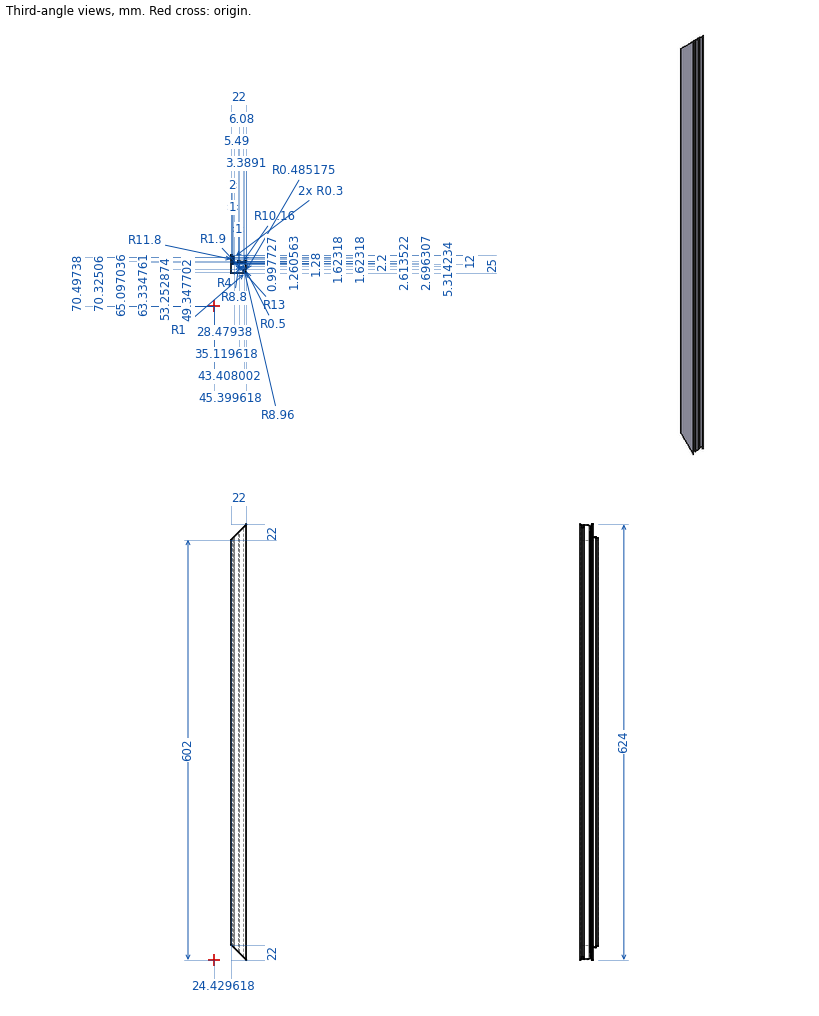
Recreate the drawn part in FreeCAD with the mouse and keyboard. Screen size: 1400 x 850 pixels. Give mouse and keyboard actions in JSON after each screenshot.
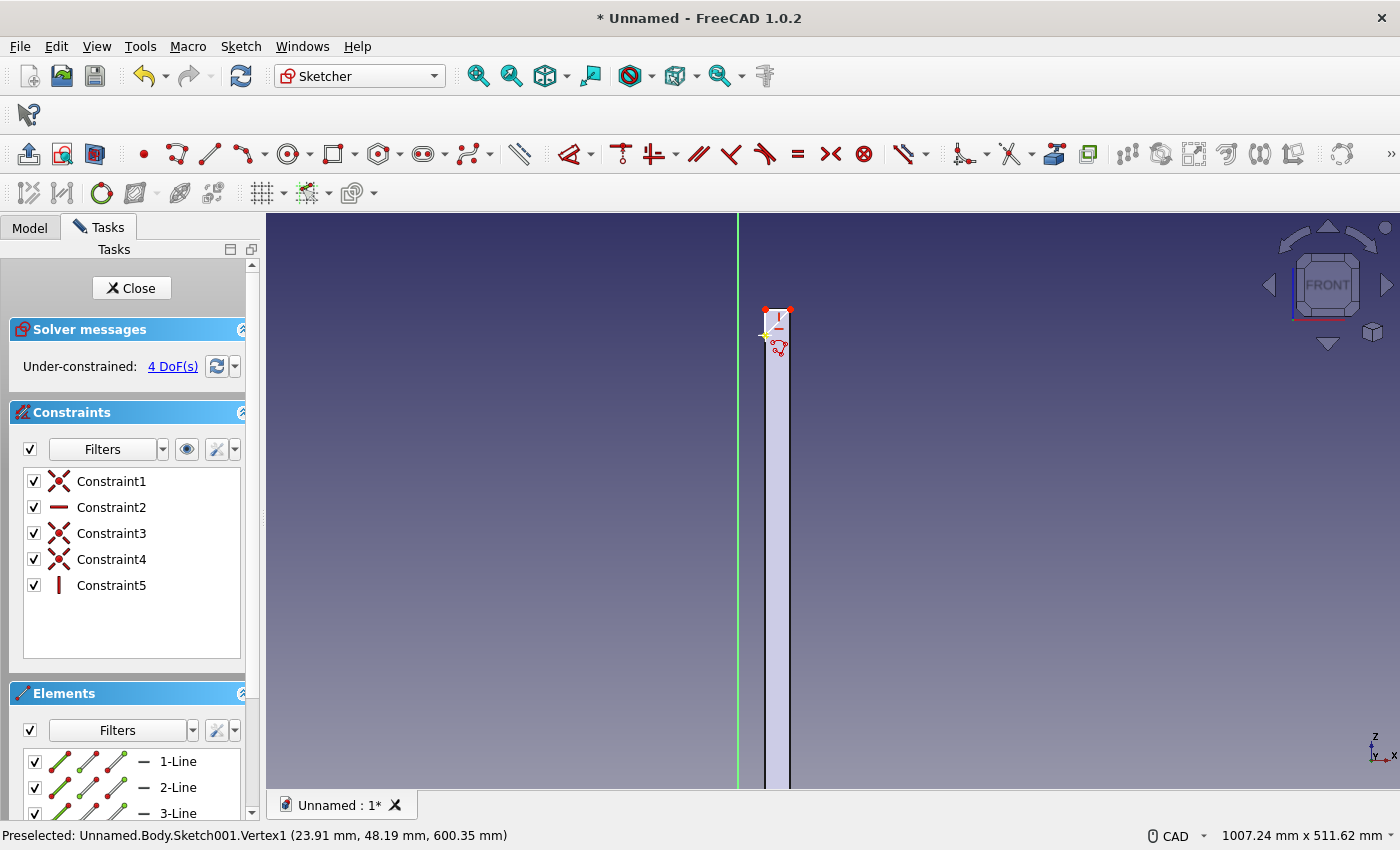
{"action": "scroll", "coordinate": [765, 308], "scroll_direction": "down", "scroll_amount": 3}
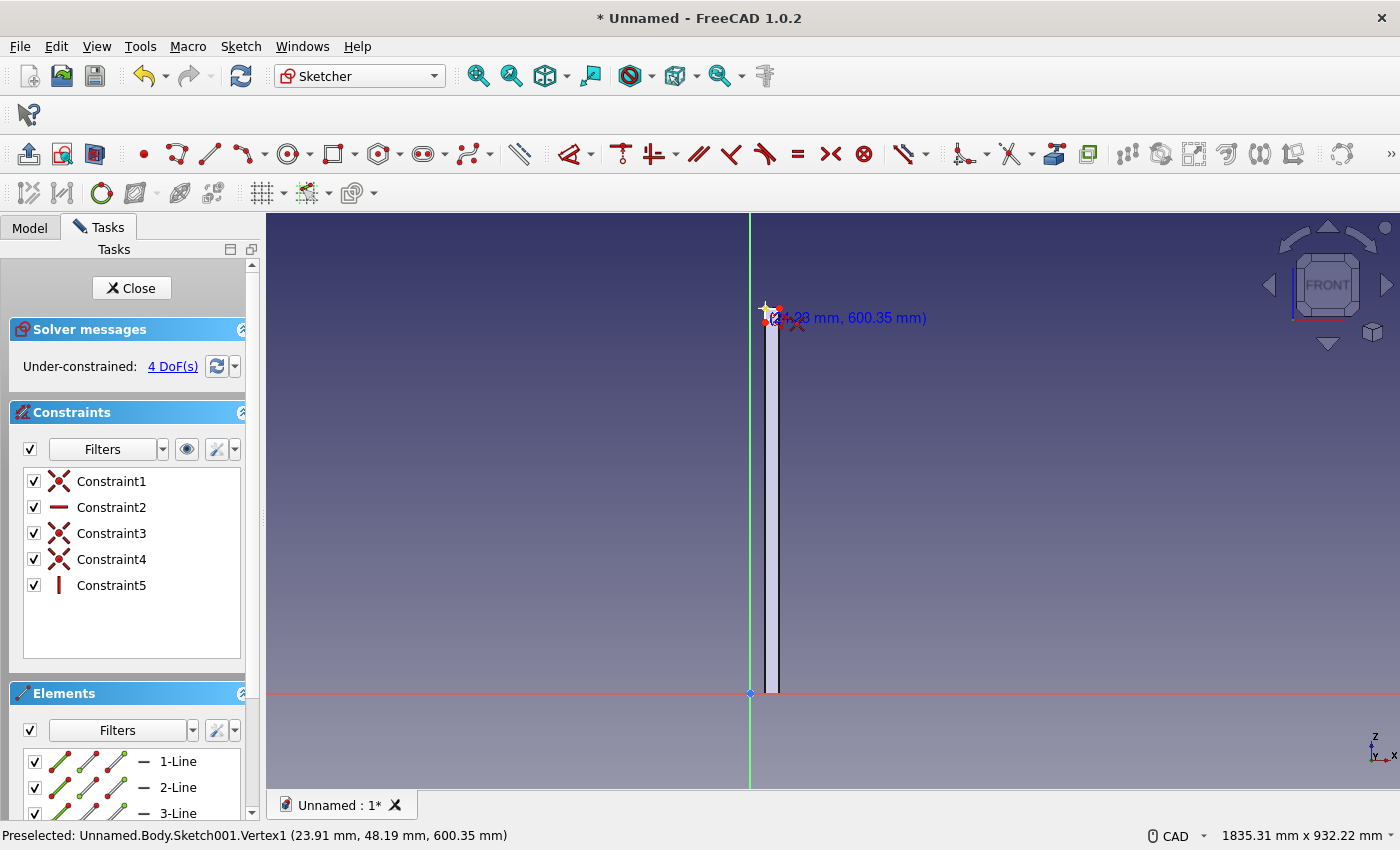
{"action": "left_click", "coordinate": [765, 694]}
{"action": "left_click", "coordinate": [779, 685]}
{"action": "left_click", "coordinate": [765, 680]}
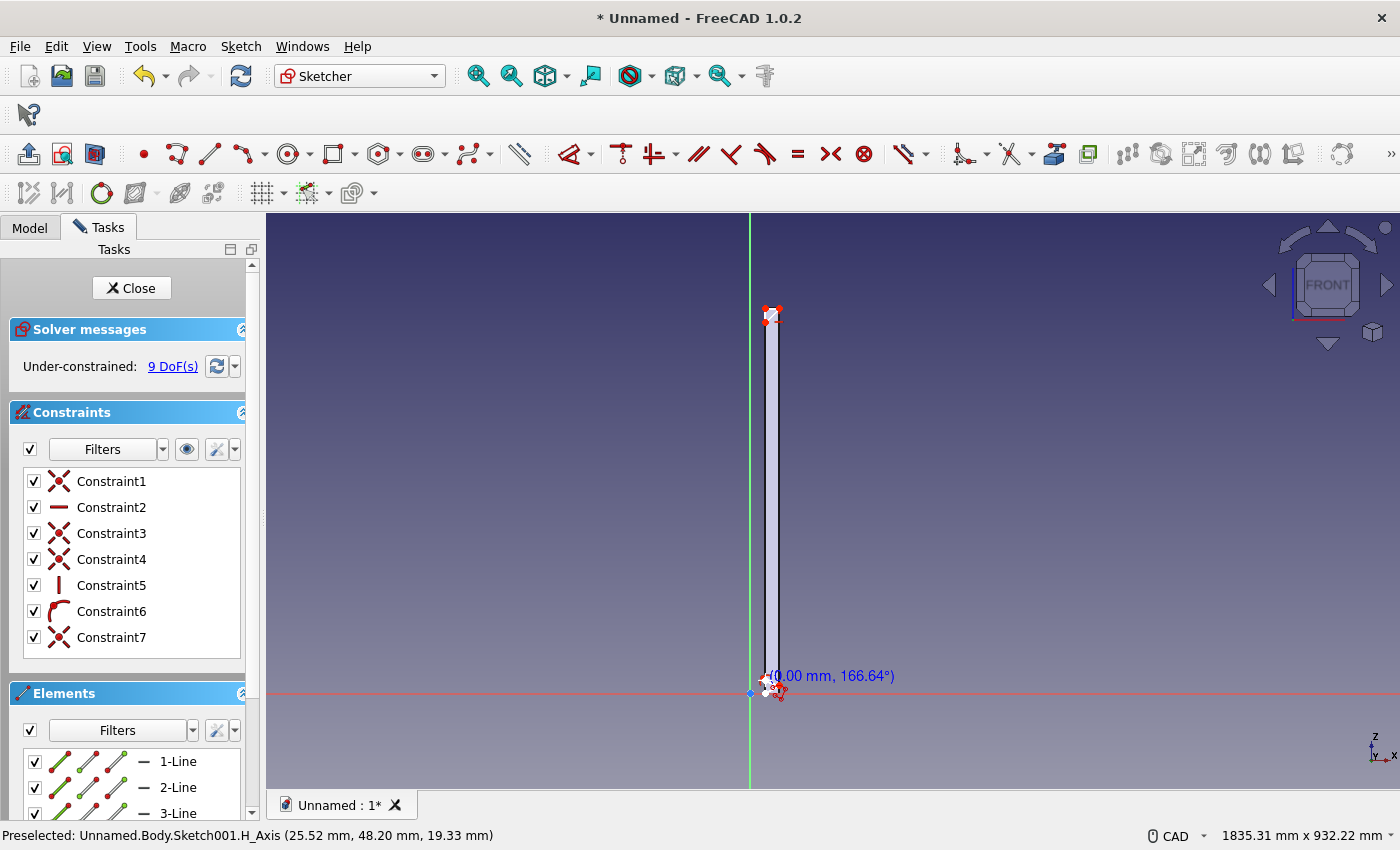
{"action": "scroll", "coordinate": [765, 694], "scroll_direction": "up", "scroll_amount": 5}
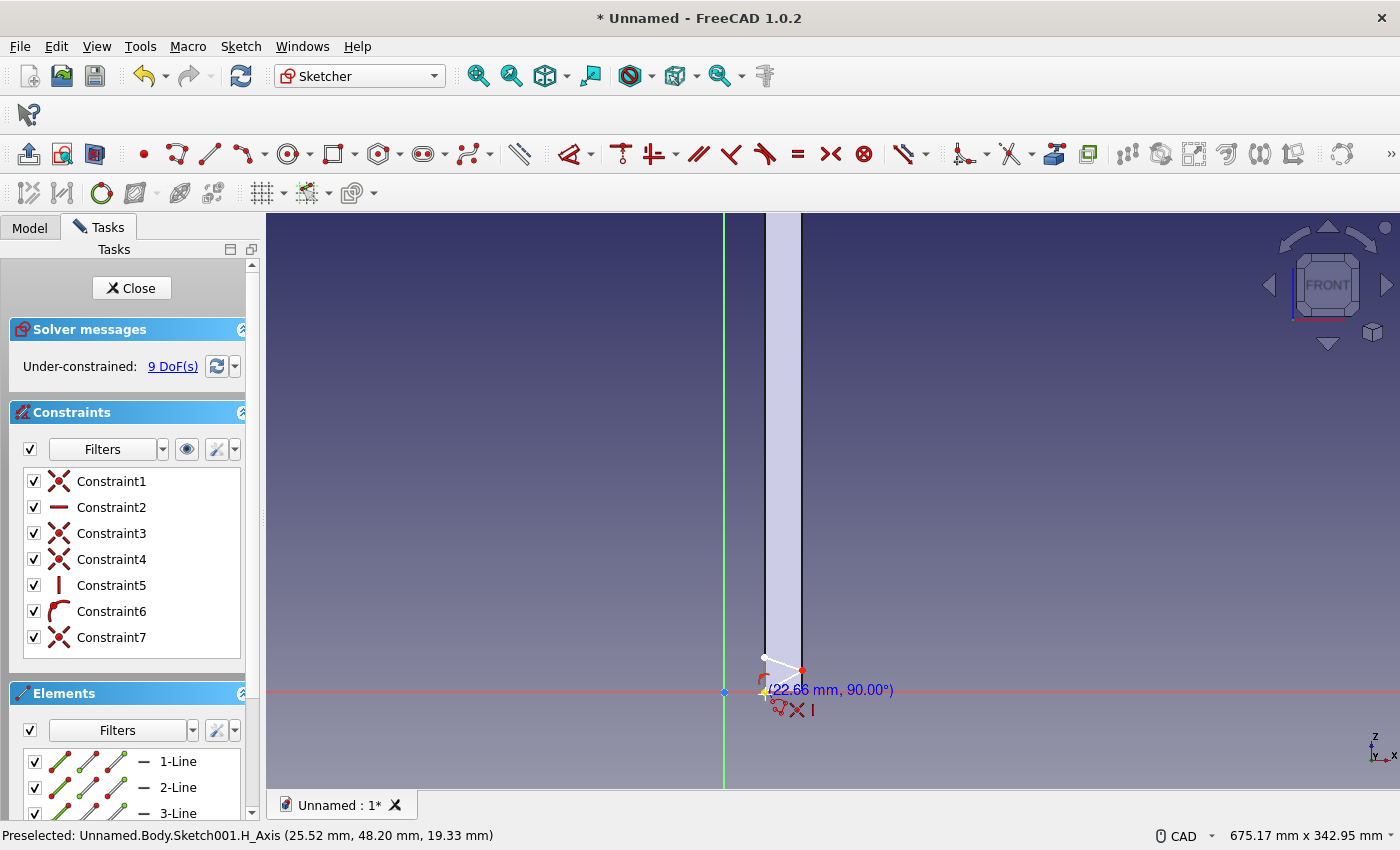
{"action": "left_click", "coordinate": [764, 692]}
{"action": "key", "text": "Escape"}
{"action": "key", "text": "Escape"}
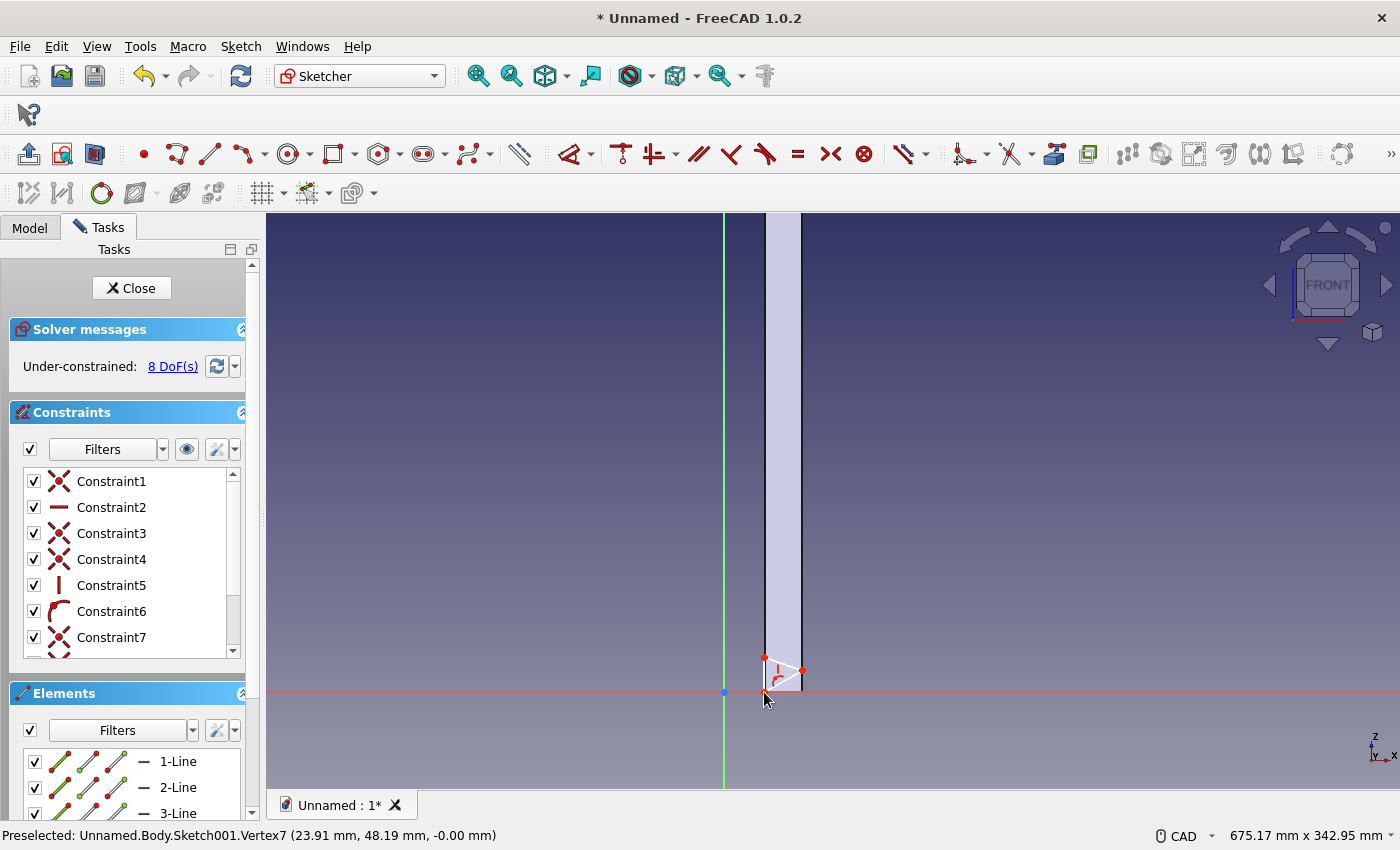
{"action": "scroll", "coordinate": [791, 677], "scroll_direction": "up", "scroll_amount": 2}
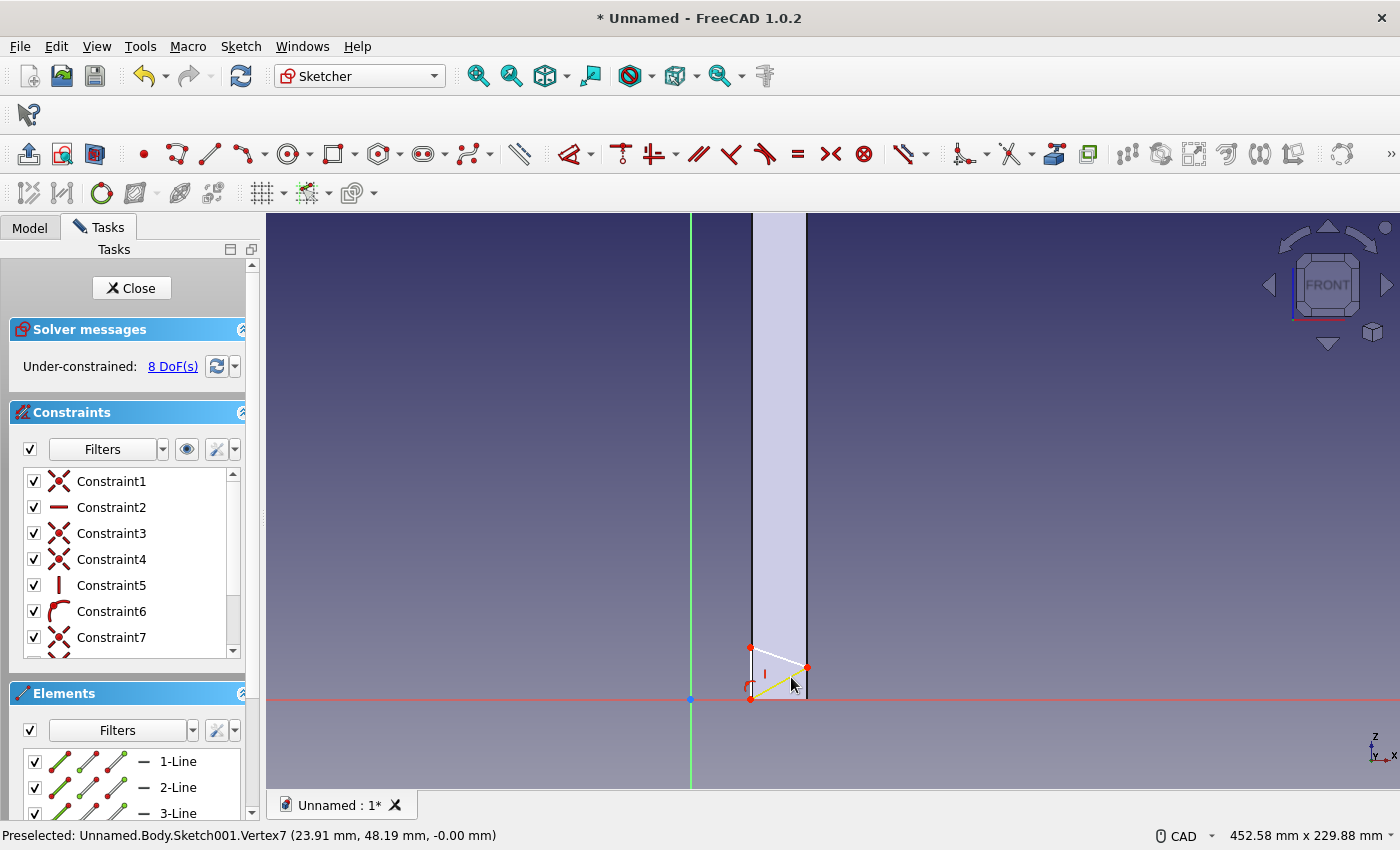
{"action": "left_click", "coordinate": [791, 677]}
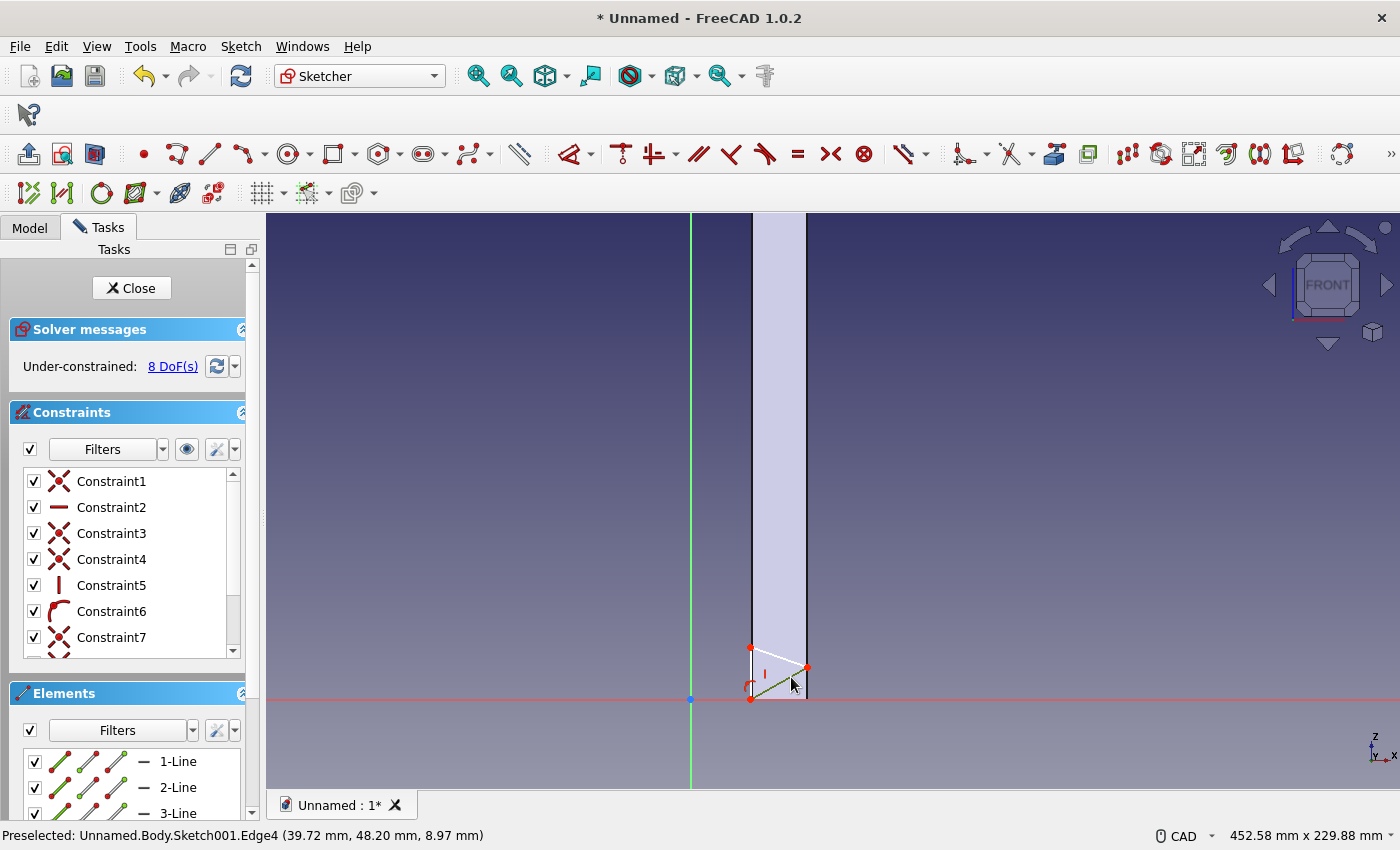
{"action": "left_click", "coordinate": [676, 154]}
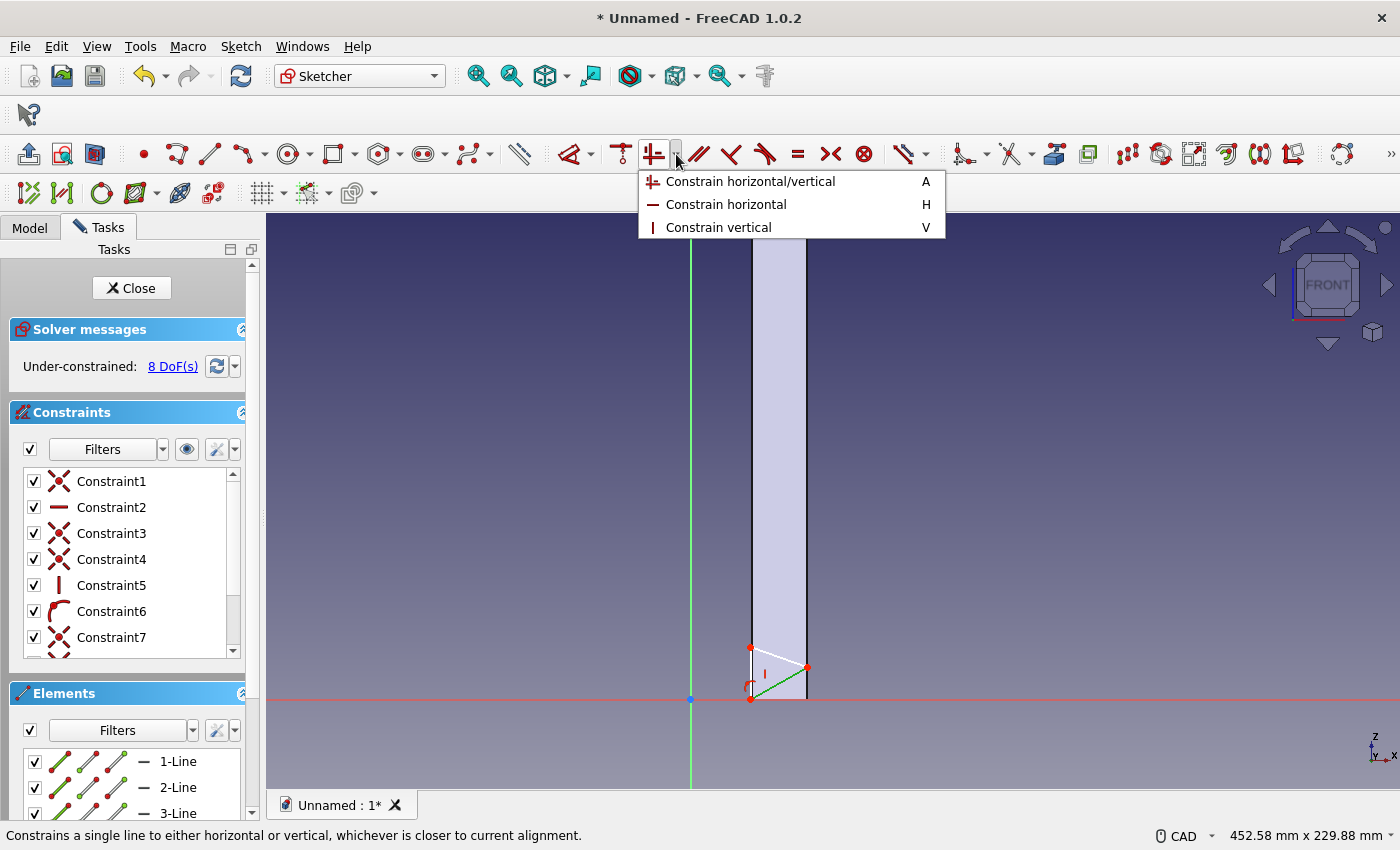
{"action": "left_click", "coordinate": [792, 204]}